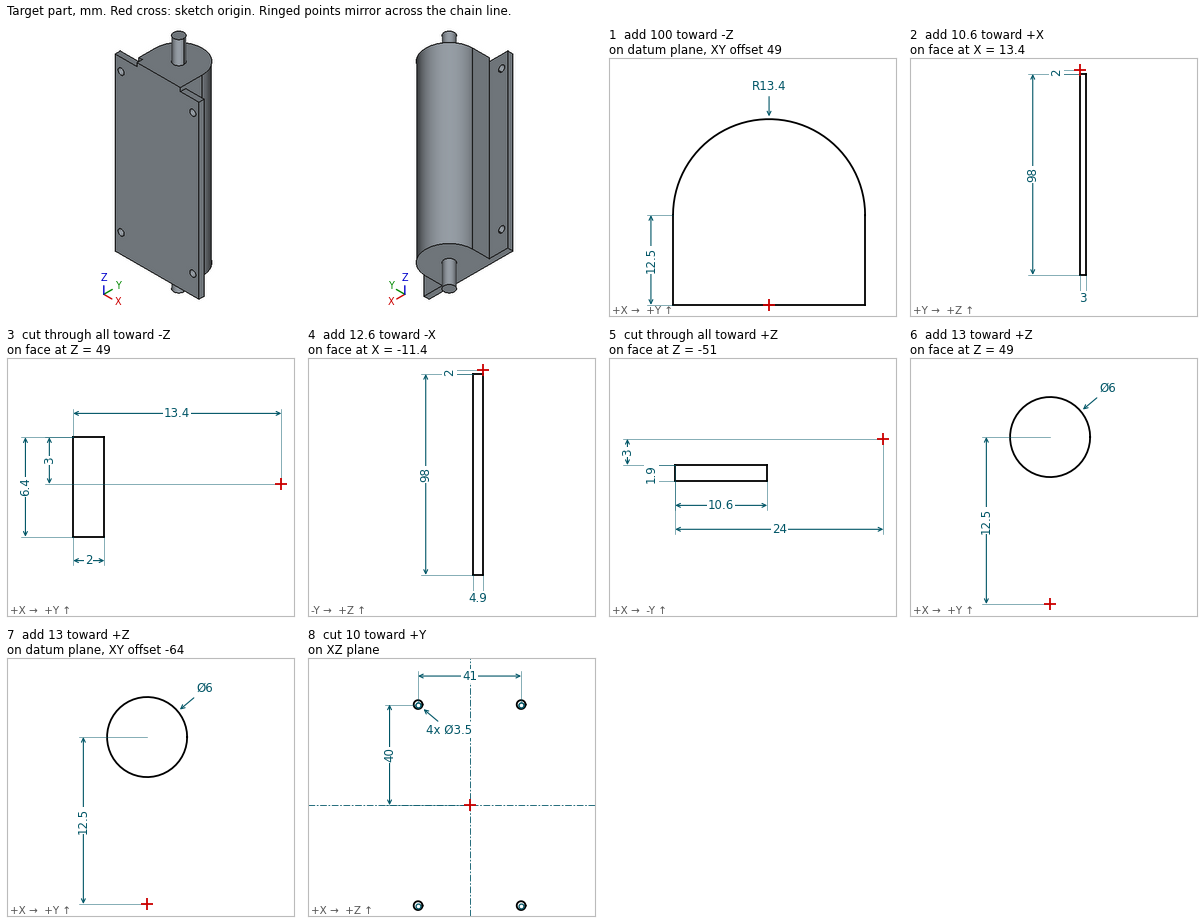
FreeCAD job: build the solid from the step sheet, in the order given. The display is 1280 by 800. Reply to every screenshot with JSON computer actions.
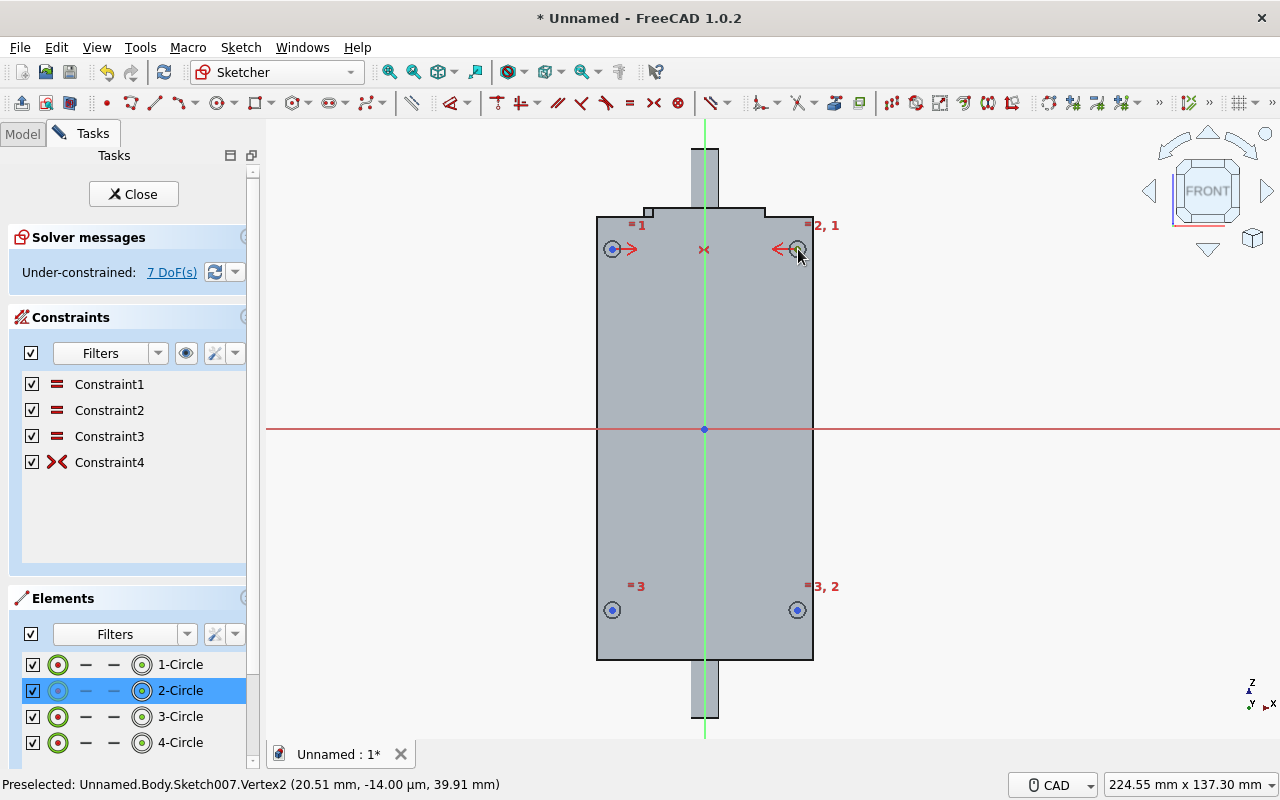
{"action": "left_click", "coordinate": [798, 610]}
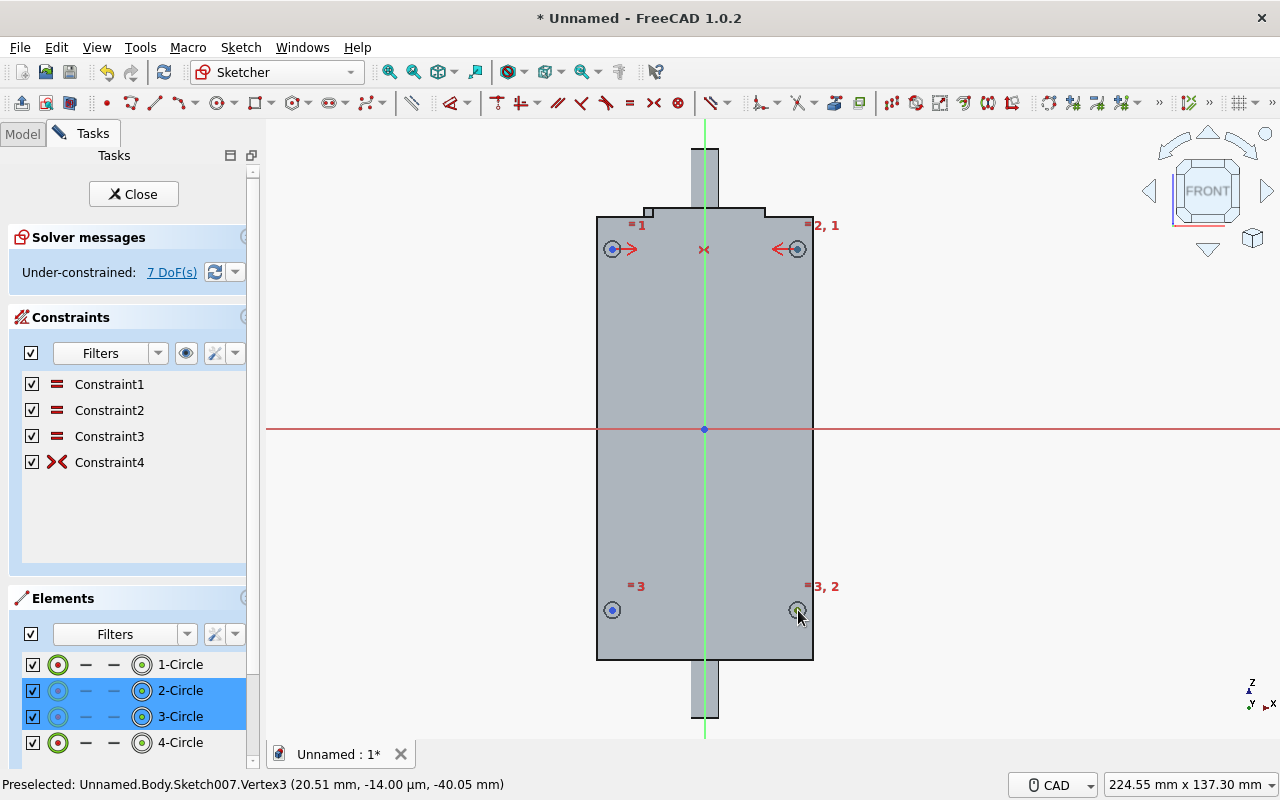
{"action": "left_click", "coordinate": [353, 429]}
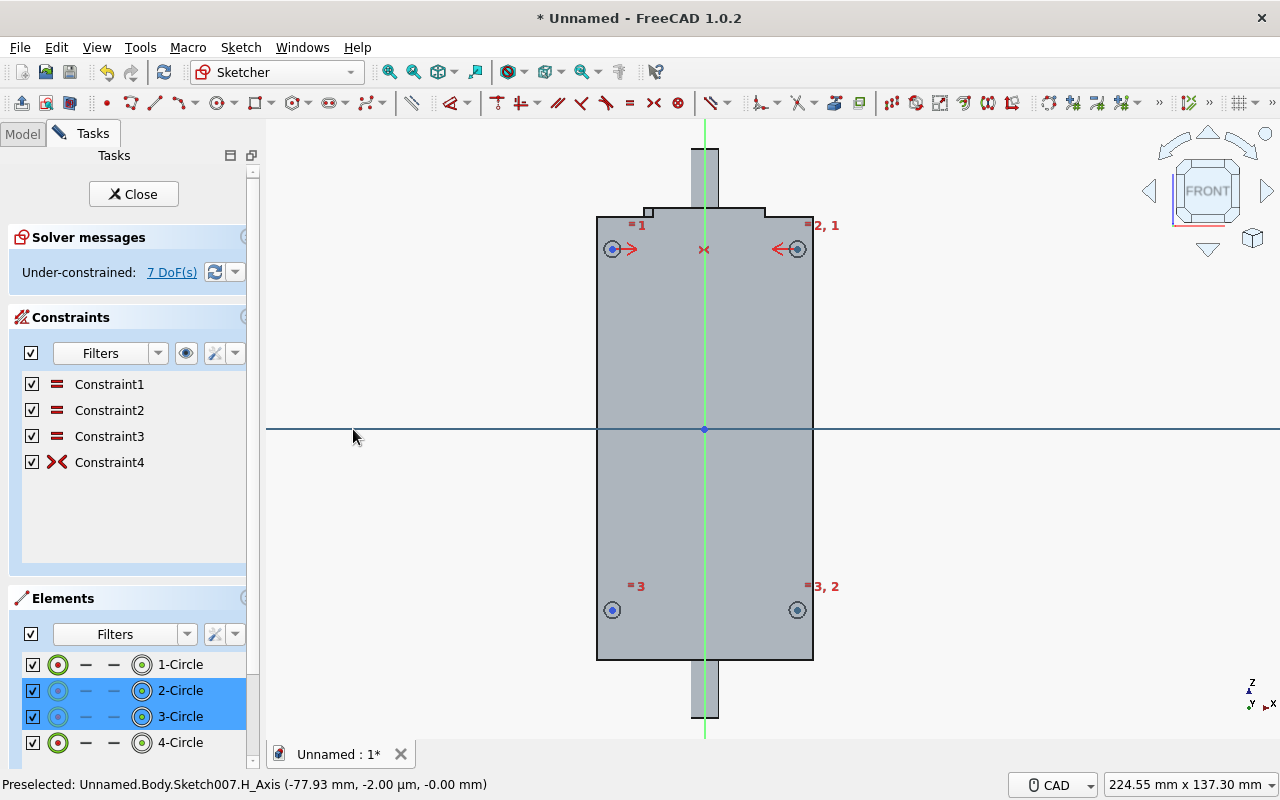
{"action": "left_click", "coordinate": [654, 104]}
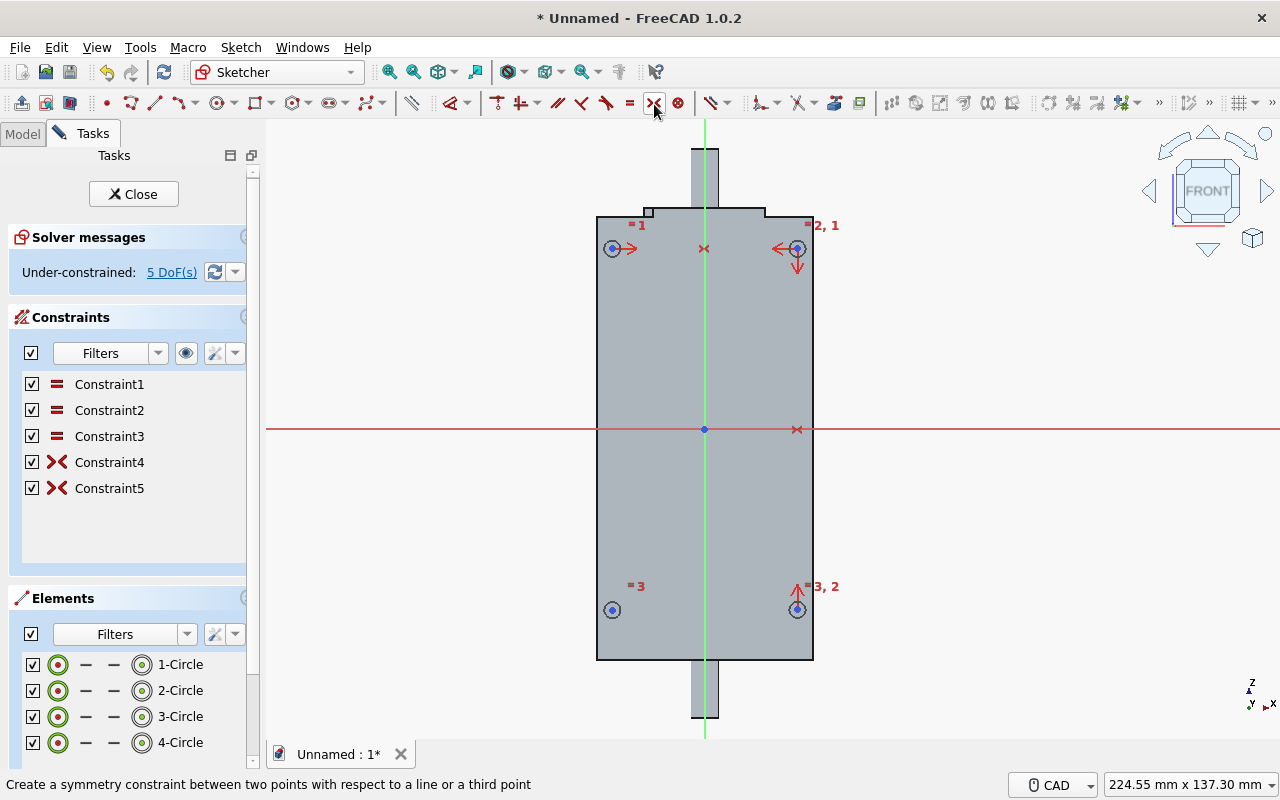
{"action": "left_click", "coordinate": [612, 249]}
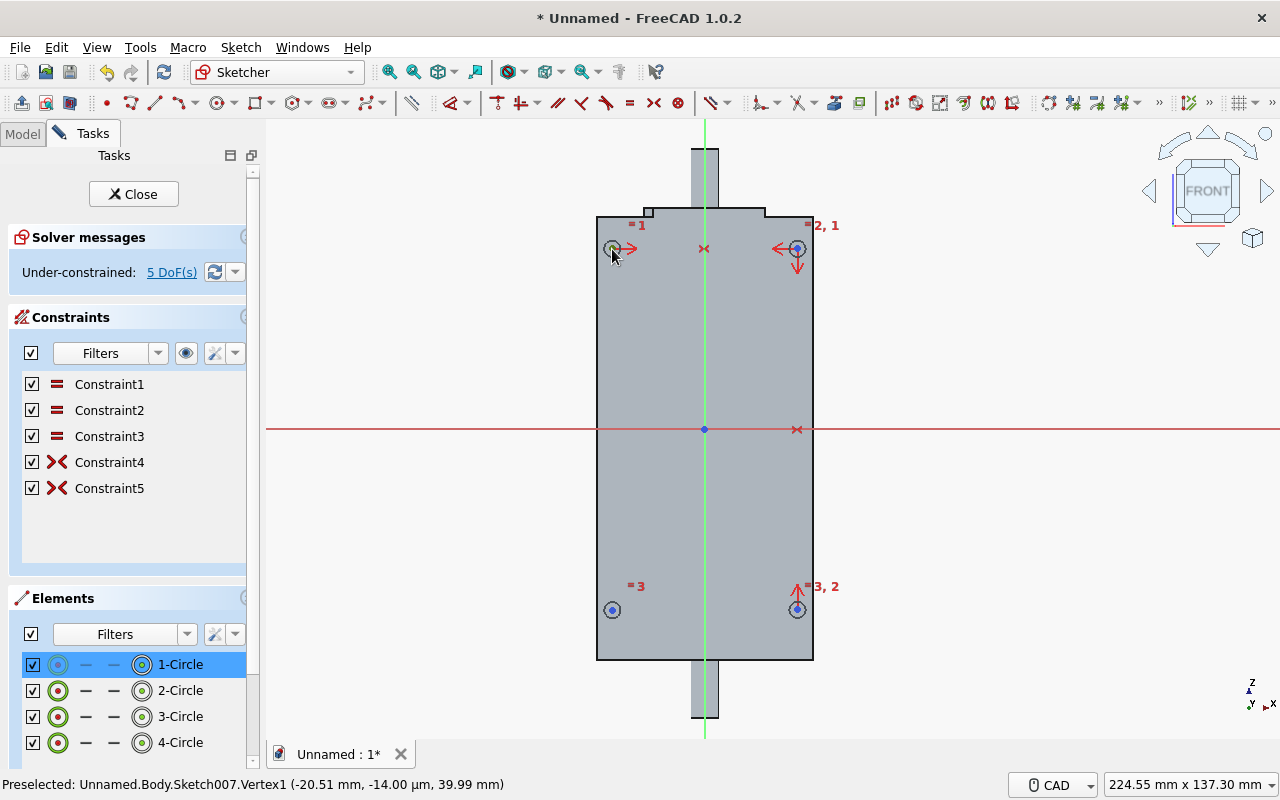
{"action": "left_click", "coordinate": [612, 610]}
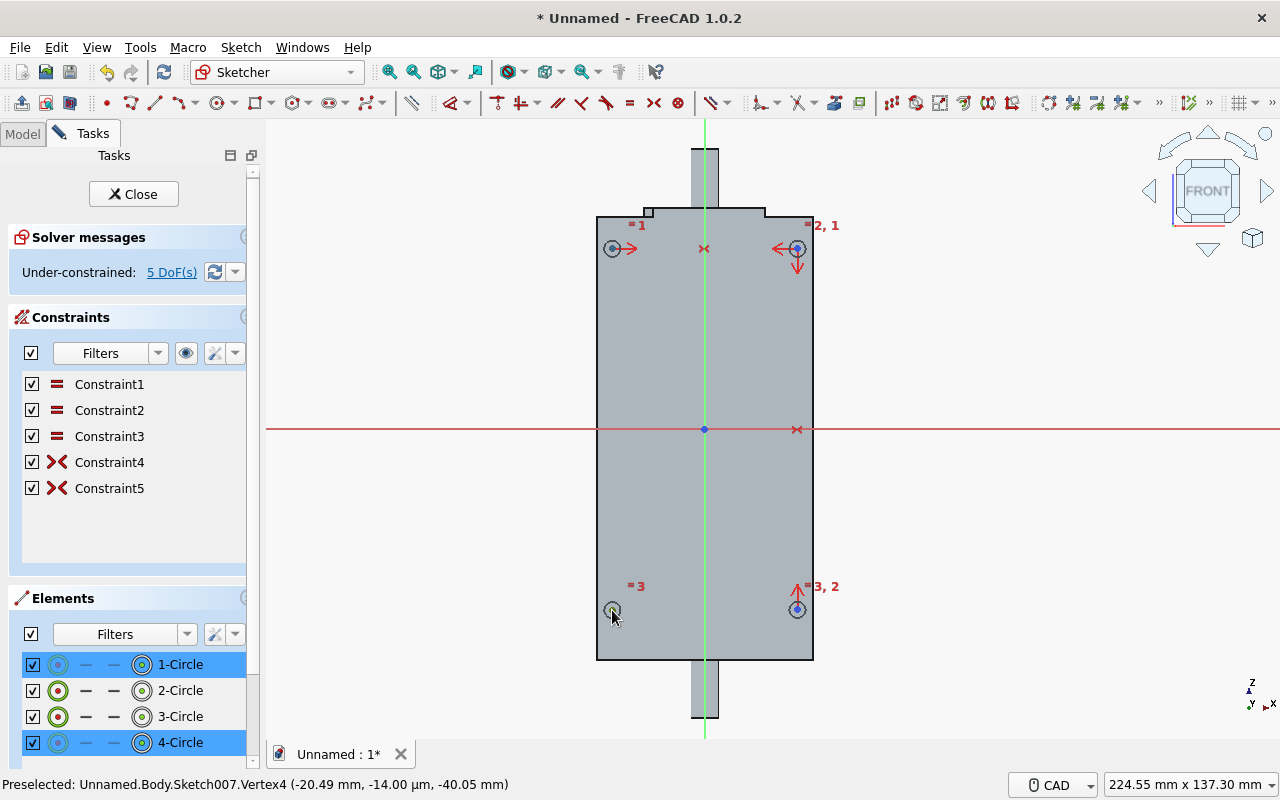
{"action": "left_click", "coordinate": [353, 429]}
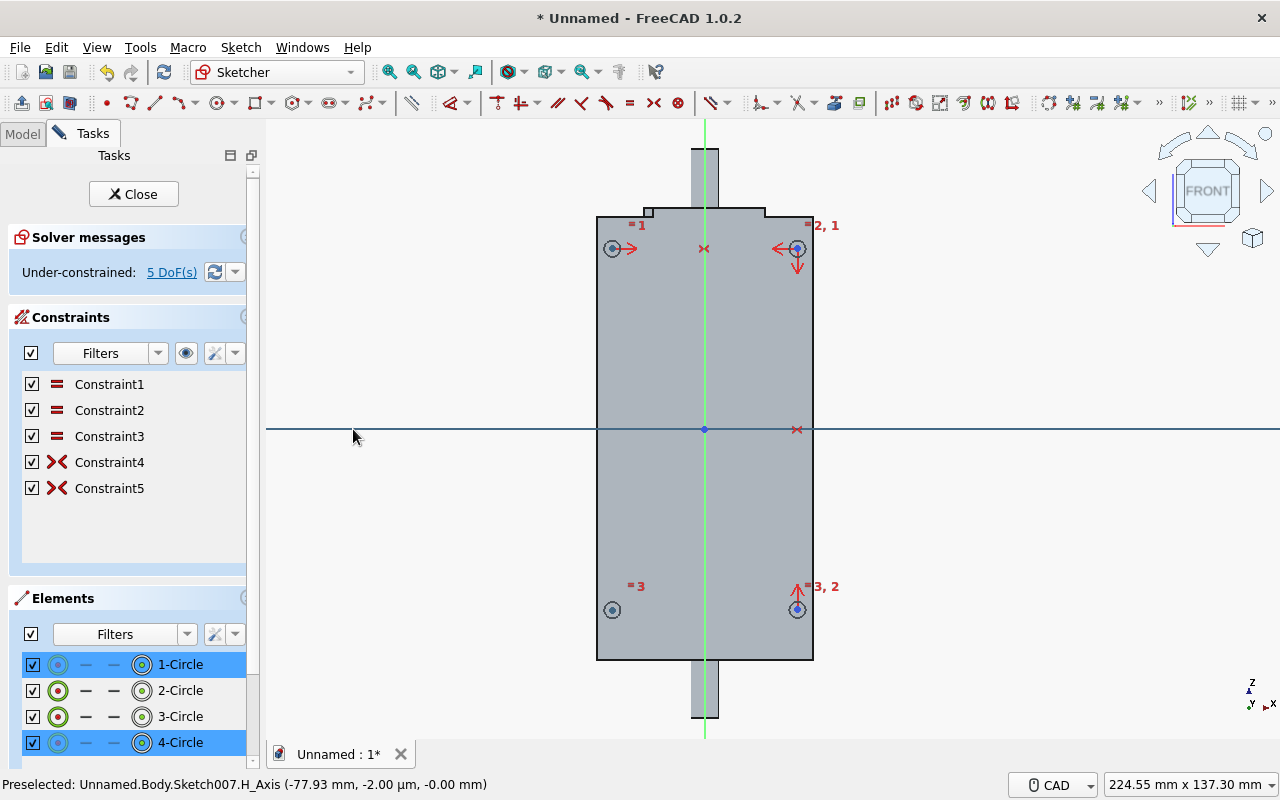
{"action": "left_click", "coordinate": [654, 104]}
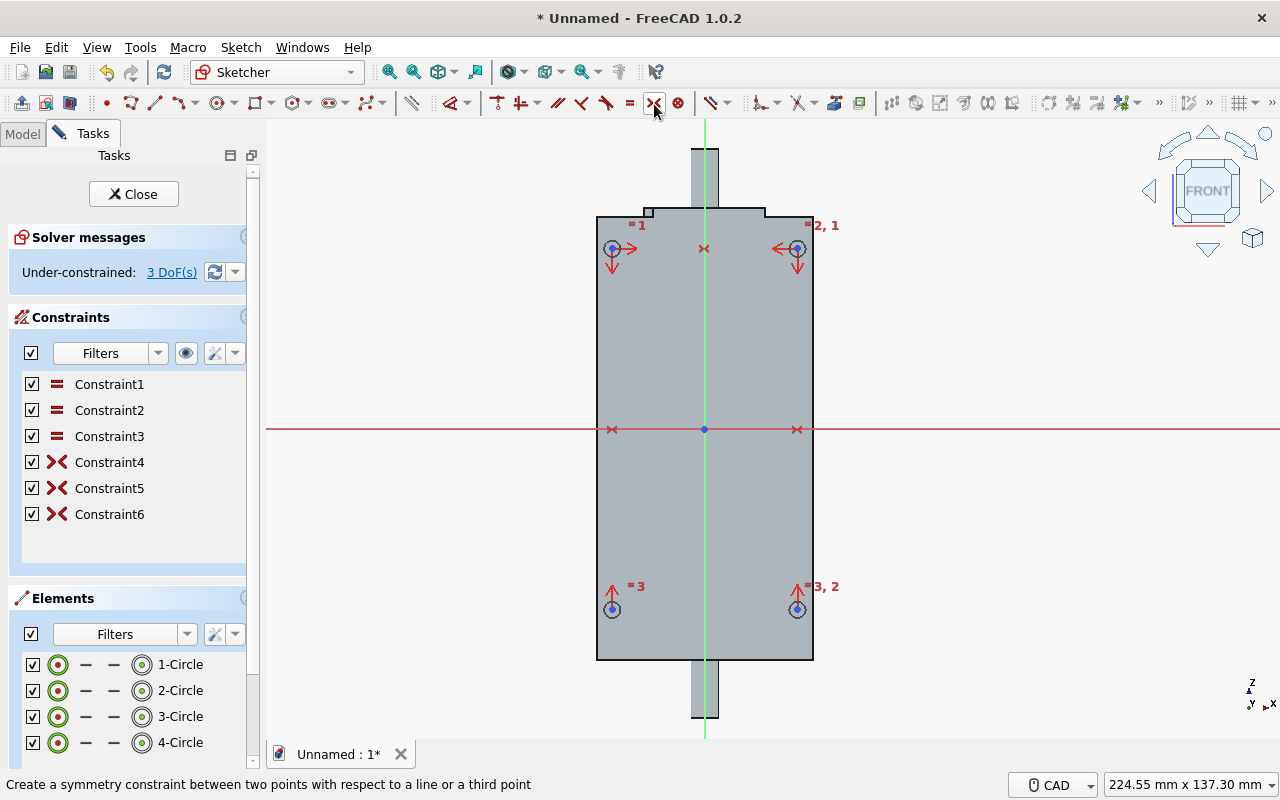
{"action": "left_click", "coordinate": [450, 104]}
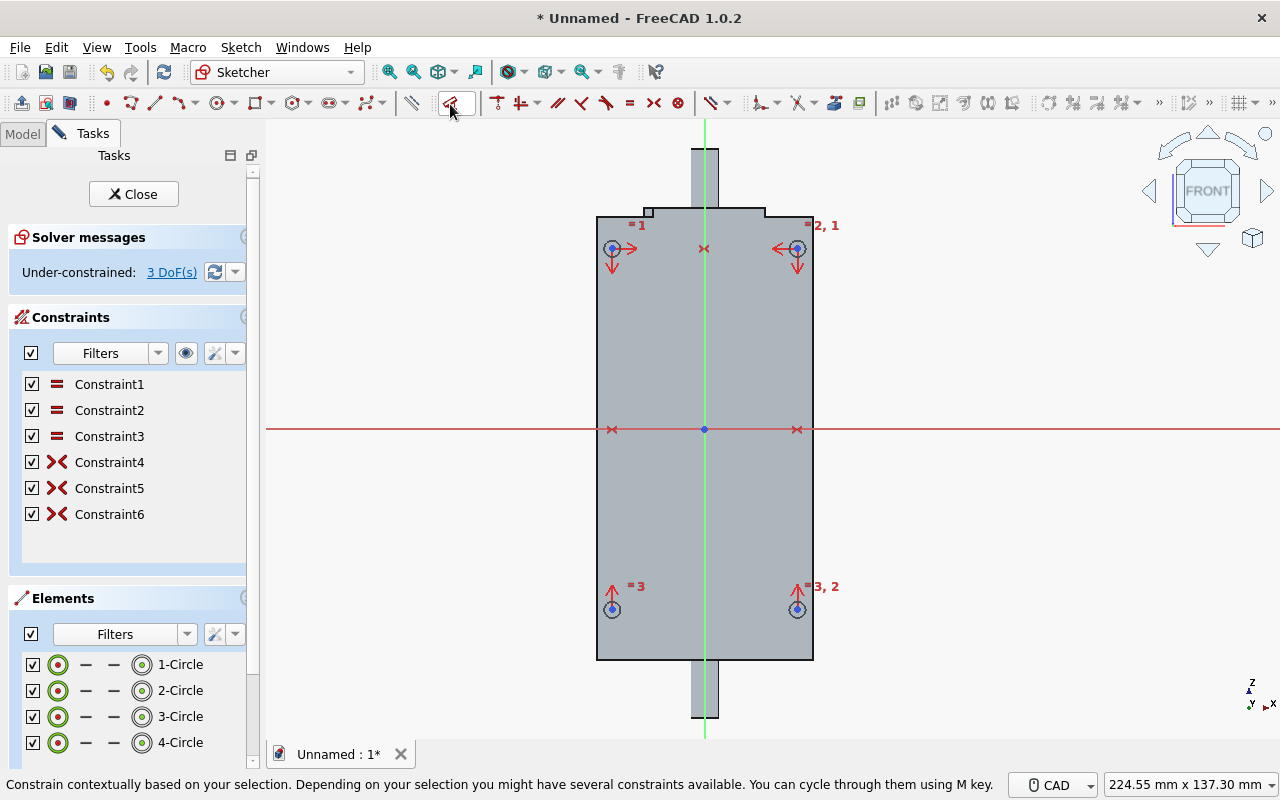
{"action": "scroll", "coordinate": [618, 243], "scroll_direction": "up", "scroll_amount": 5}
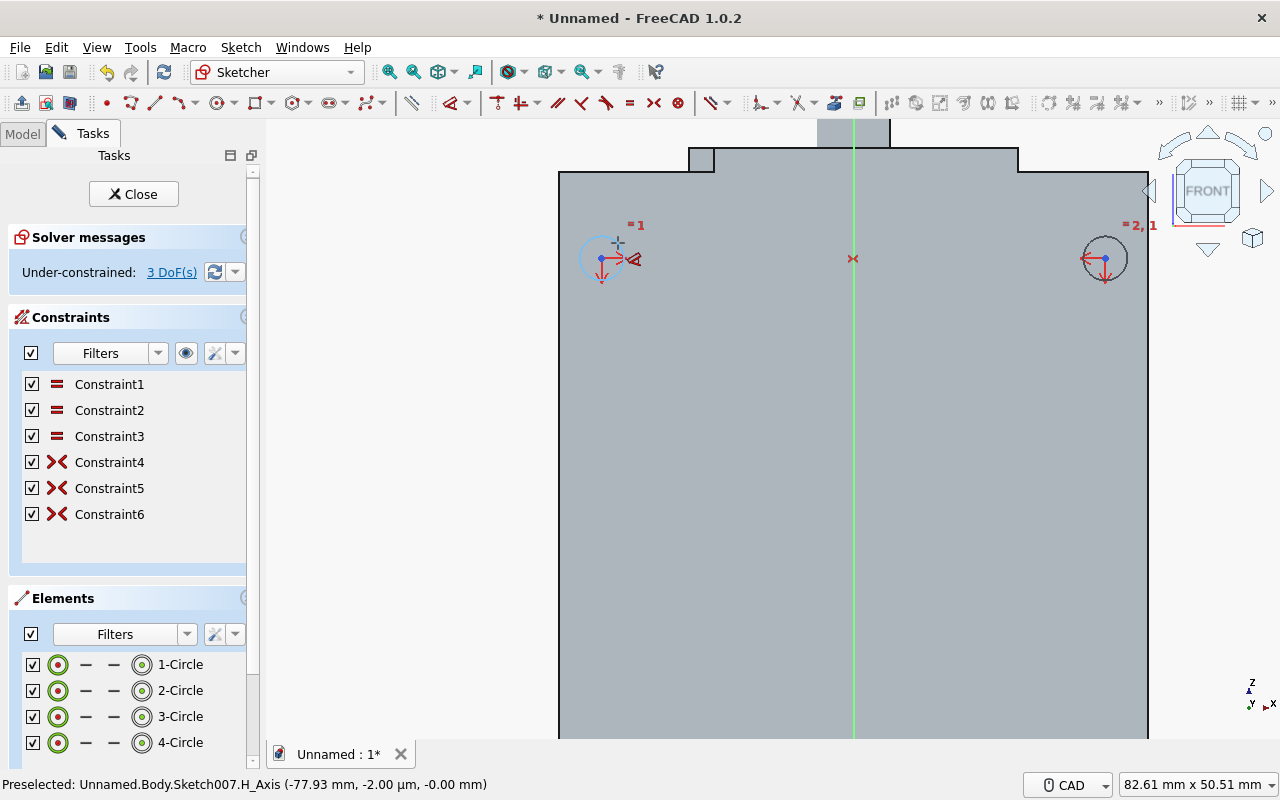
{"action": "left_click", "coordinate": [617, 243]}
{"action": "left_click", "coordinate": [639, 220]}